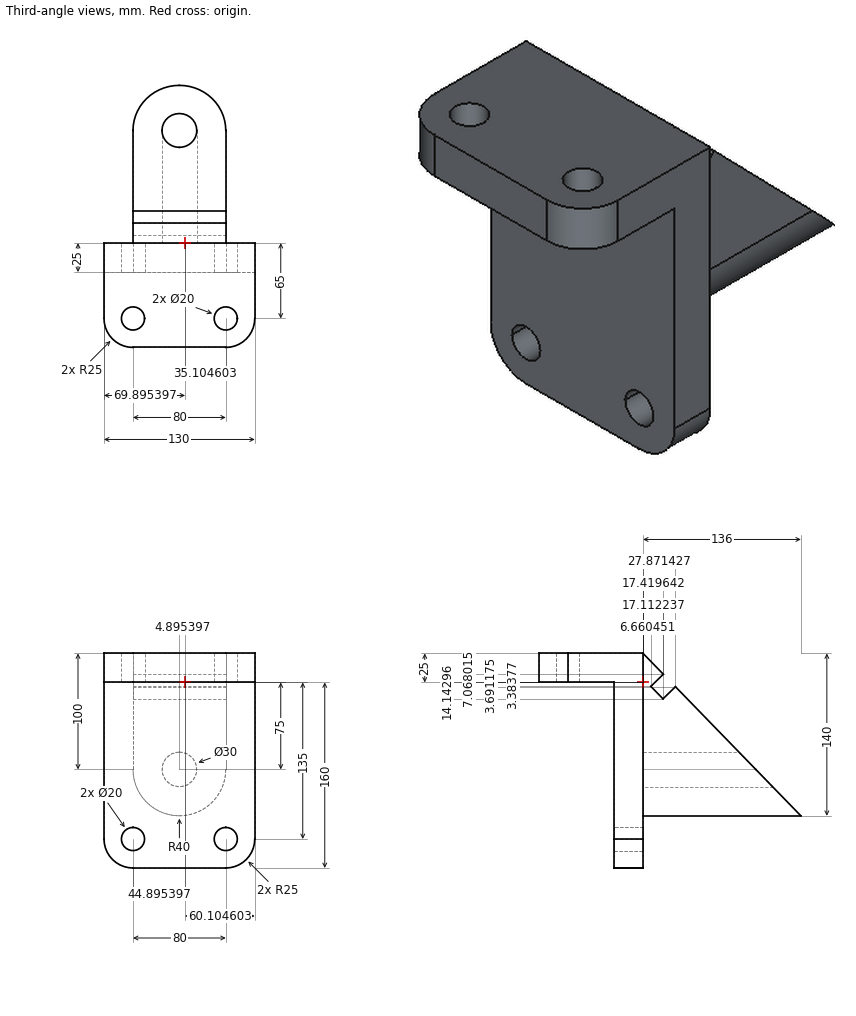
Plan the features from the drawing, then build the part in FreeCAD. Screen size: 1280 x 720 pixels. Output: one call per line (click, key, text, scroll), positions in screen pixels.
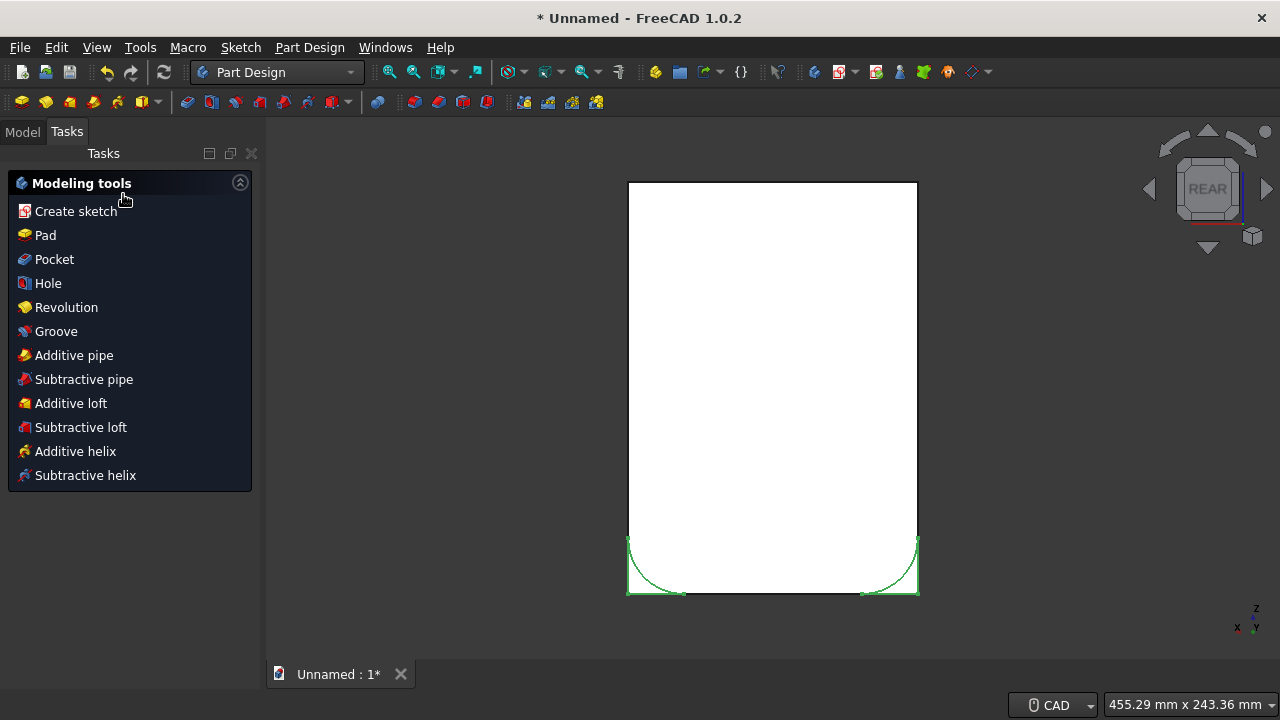
click(188, 102)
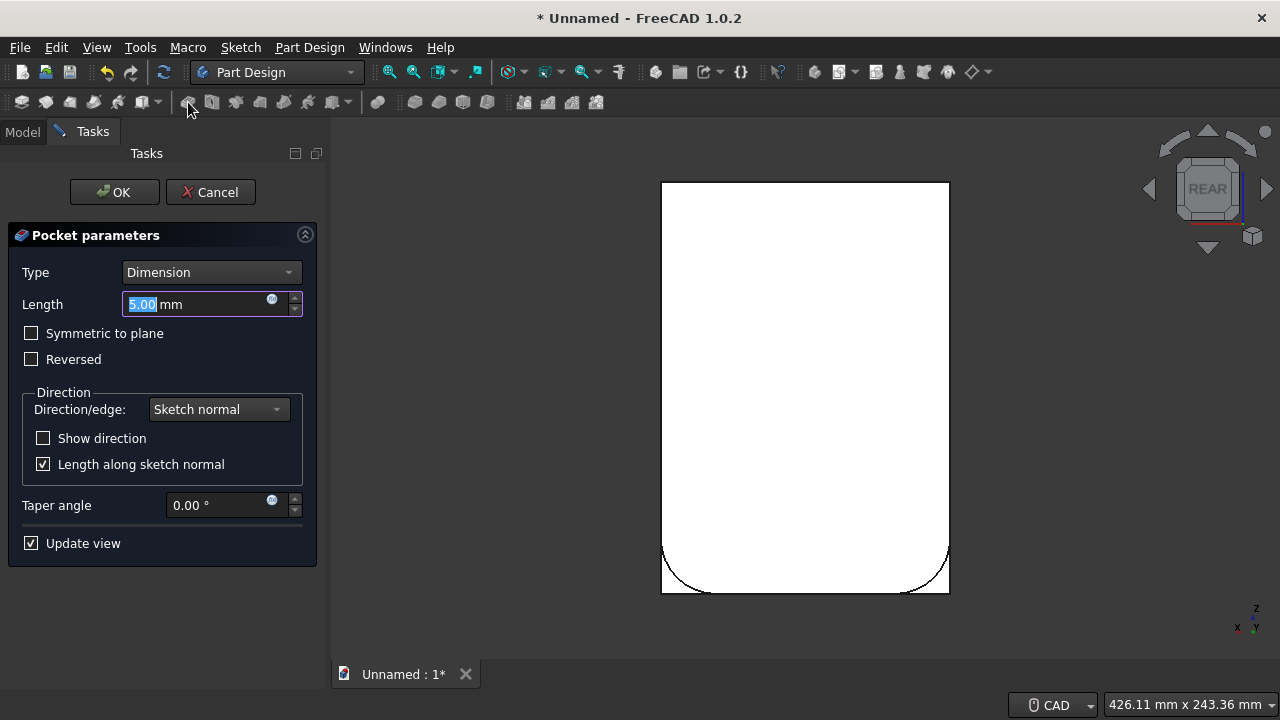
text(160)
key(Tab)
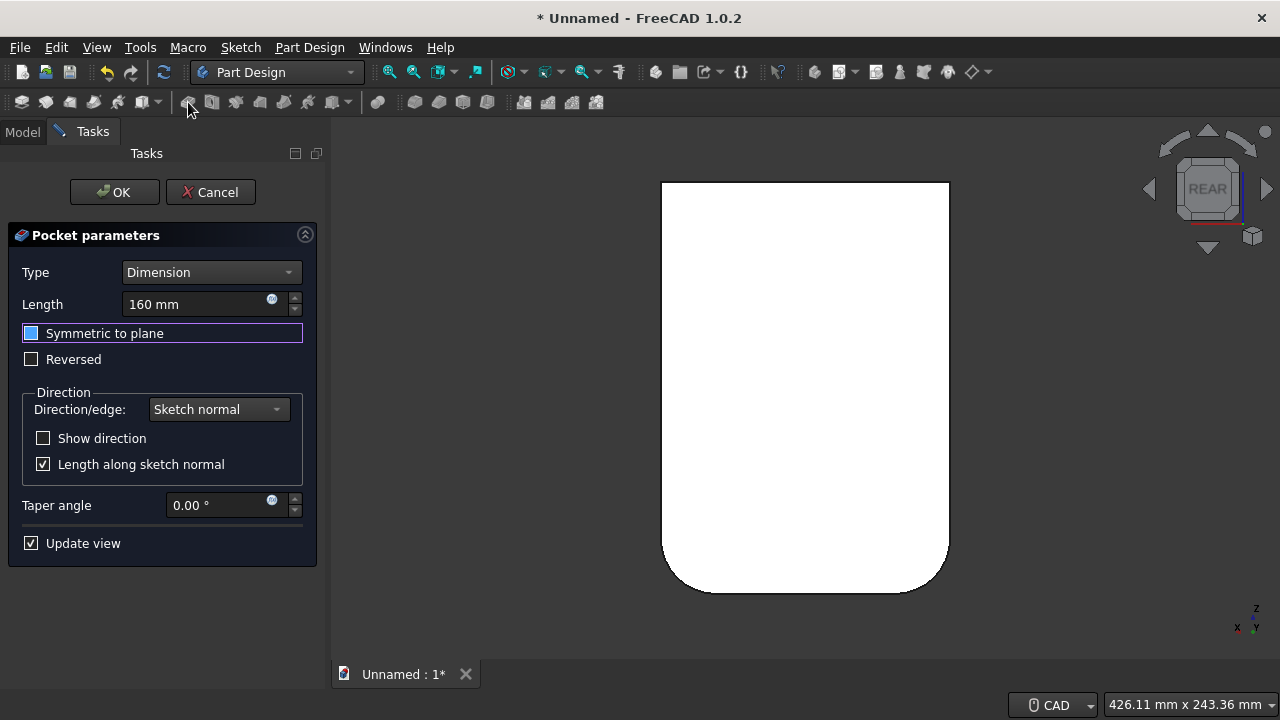
click(115, 192)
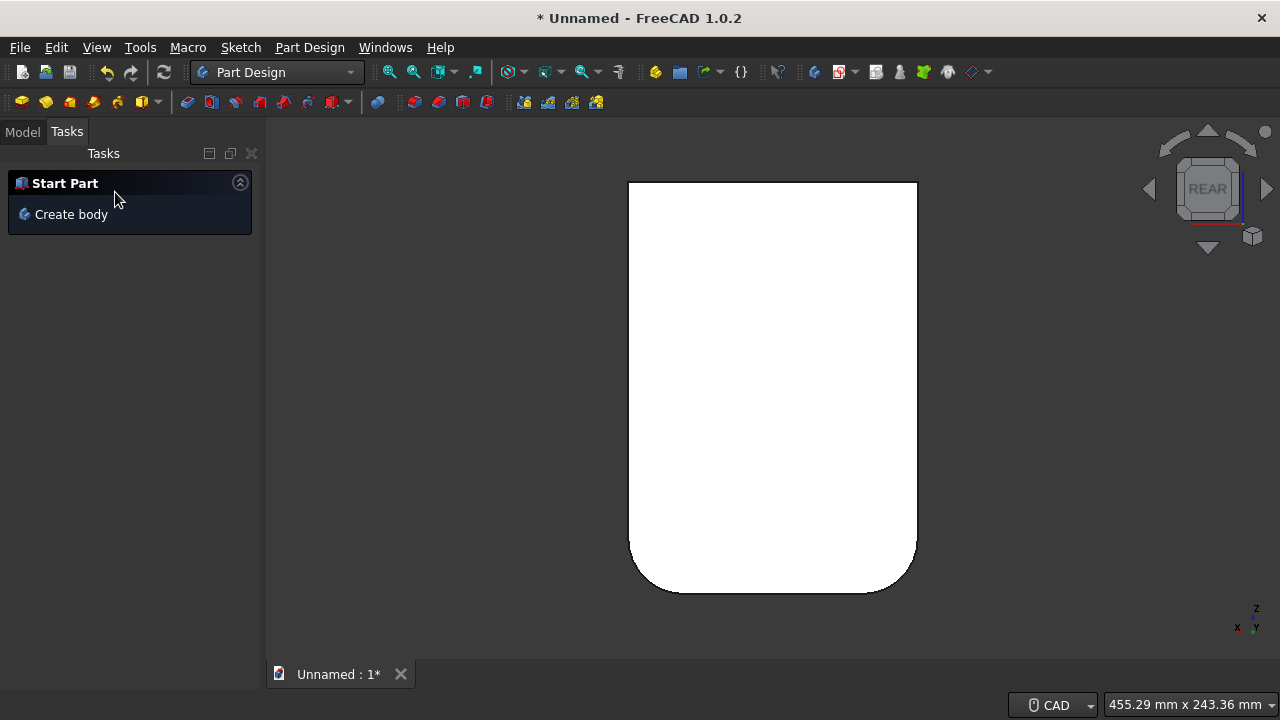
click(773, 328)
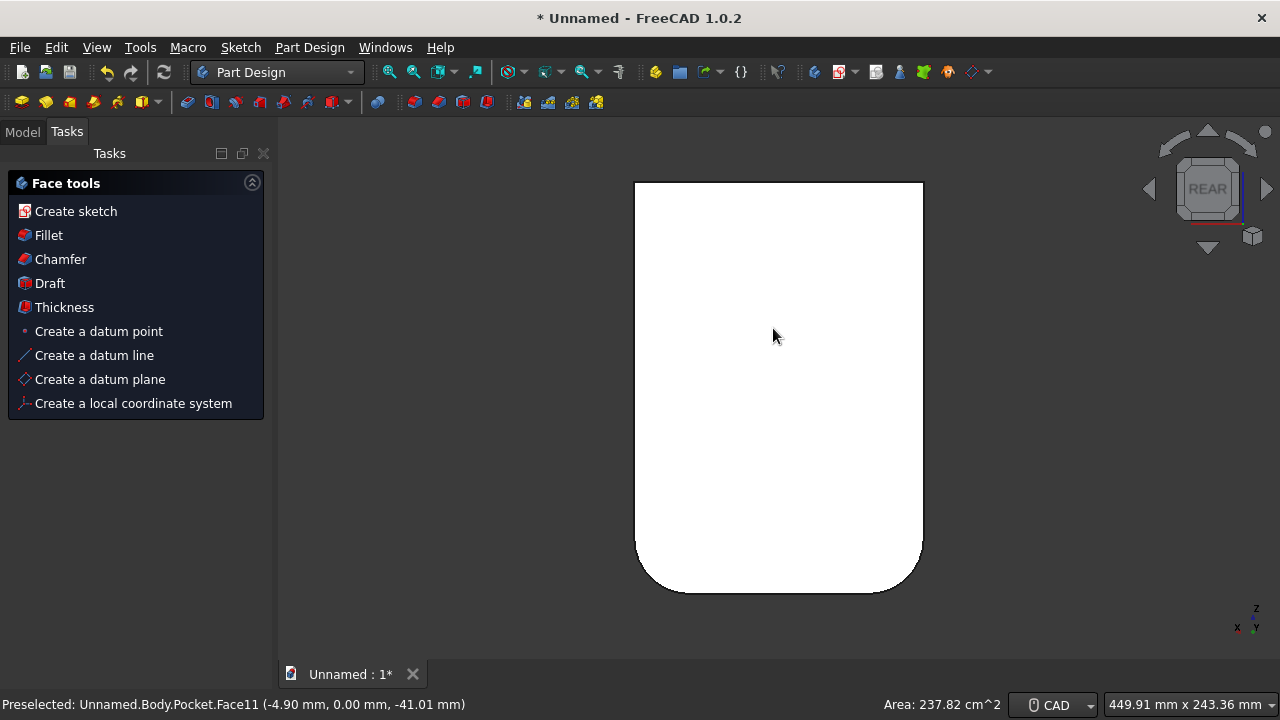
click(840, 72)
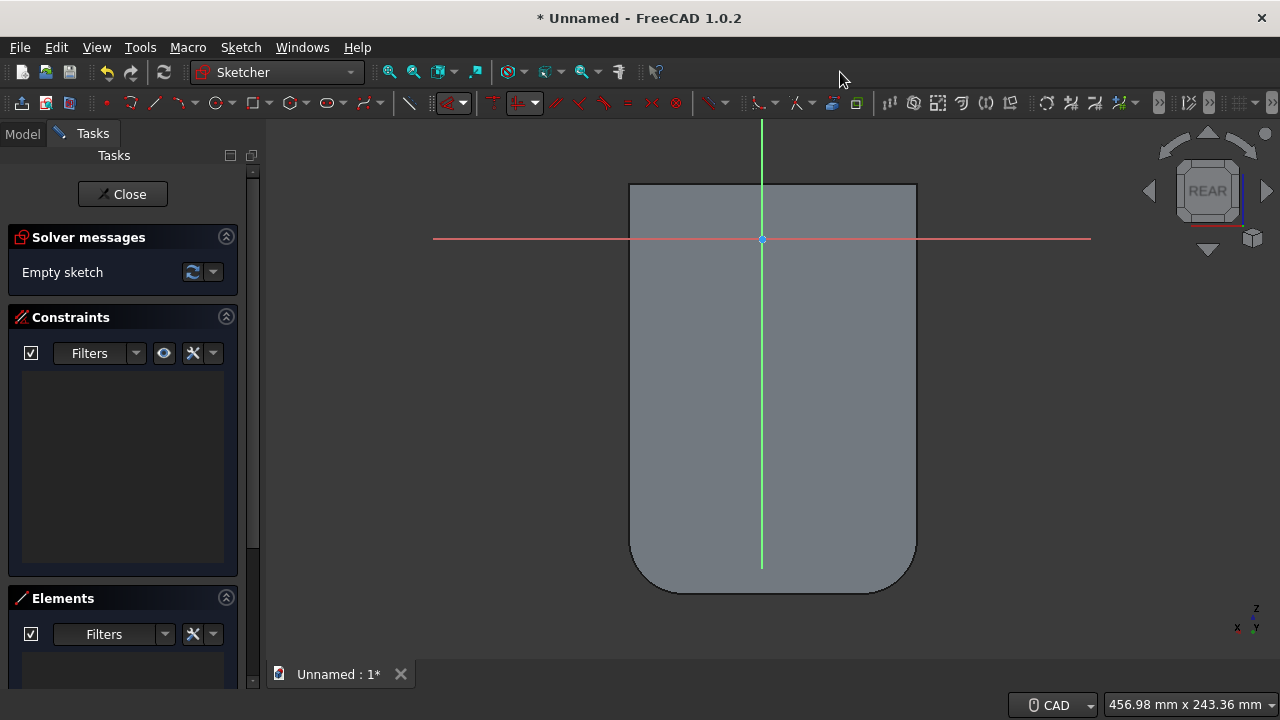
click(216, 104)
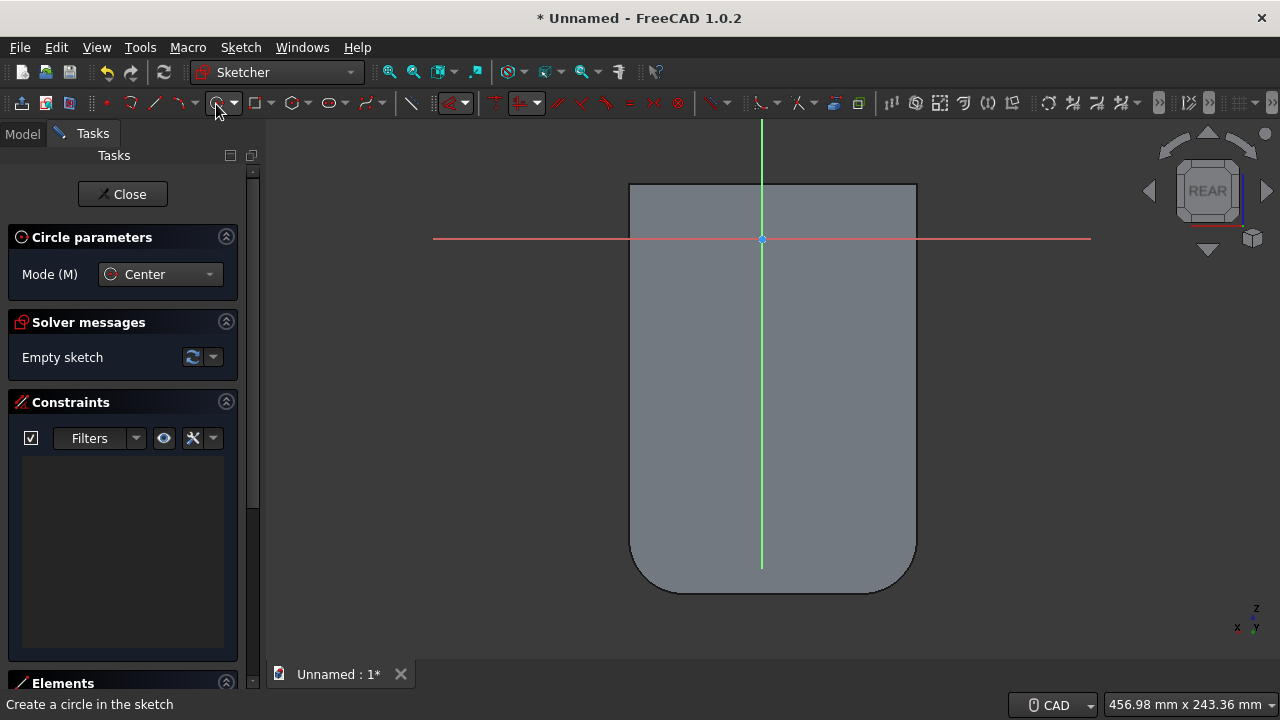
click(862, 539)
click(877, 523)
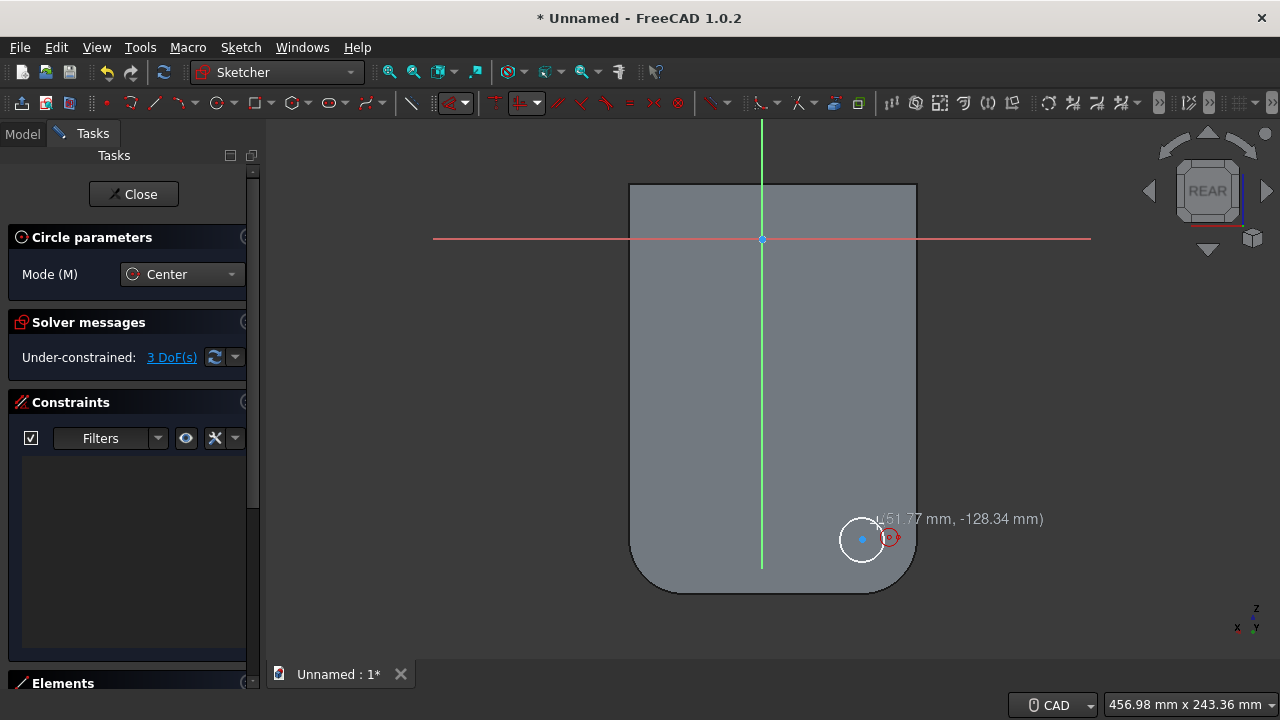
click(684, 539)
click(700, 523)
key(Escape)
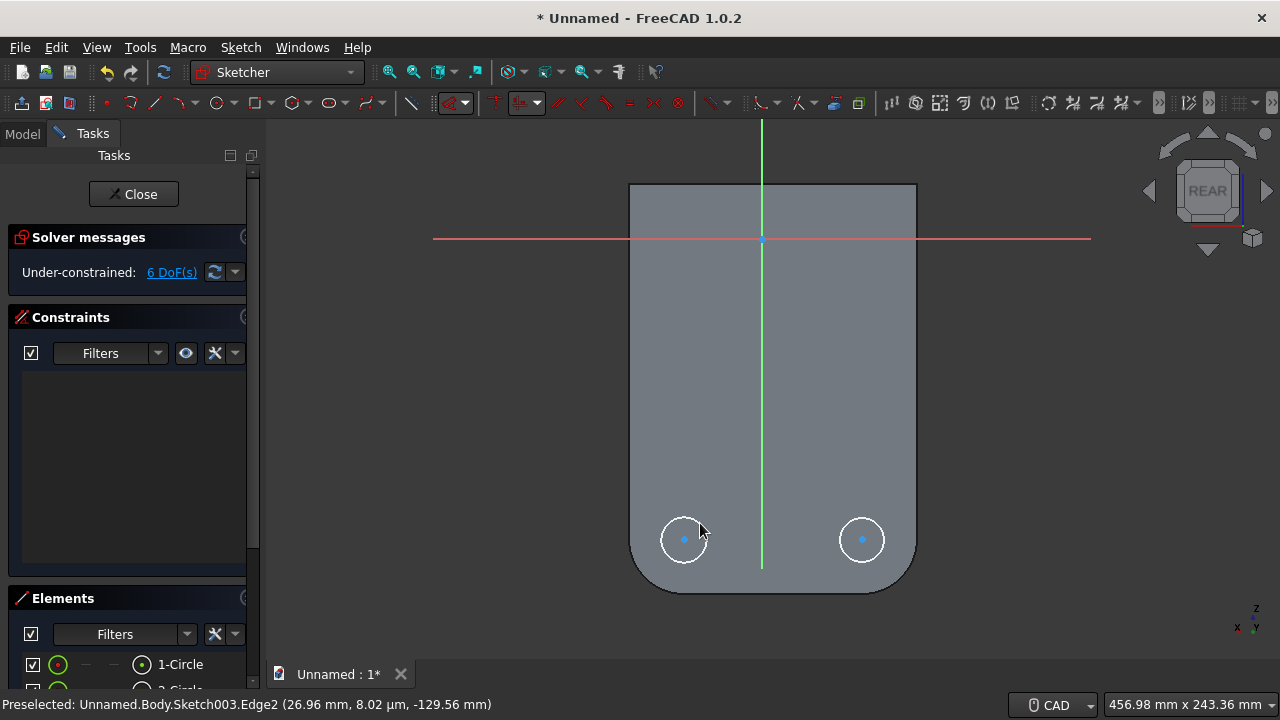
click(877, 524)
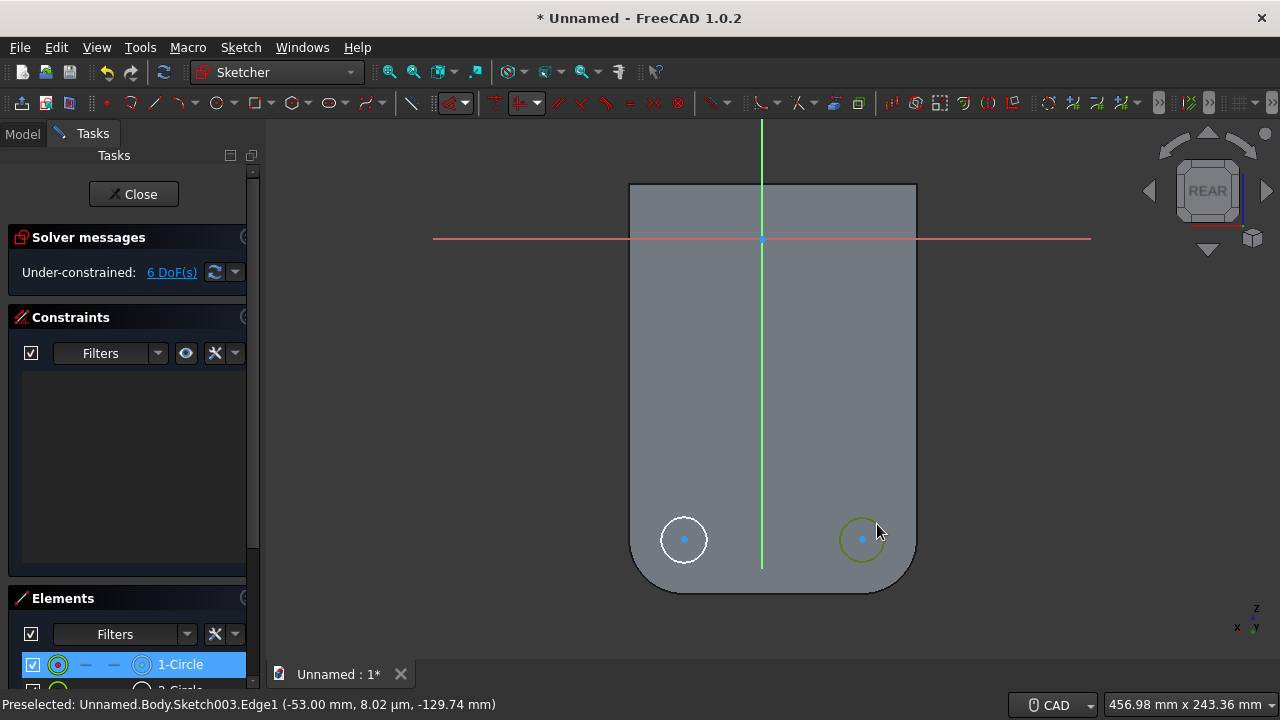
click(700, 524)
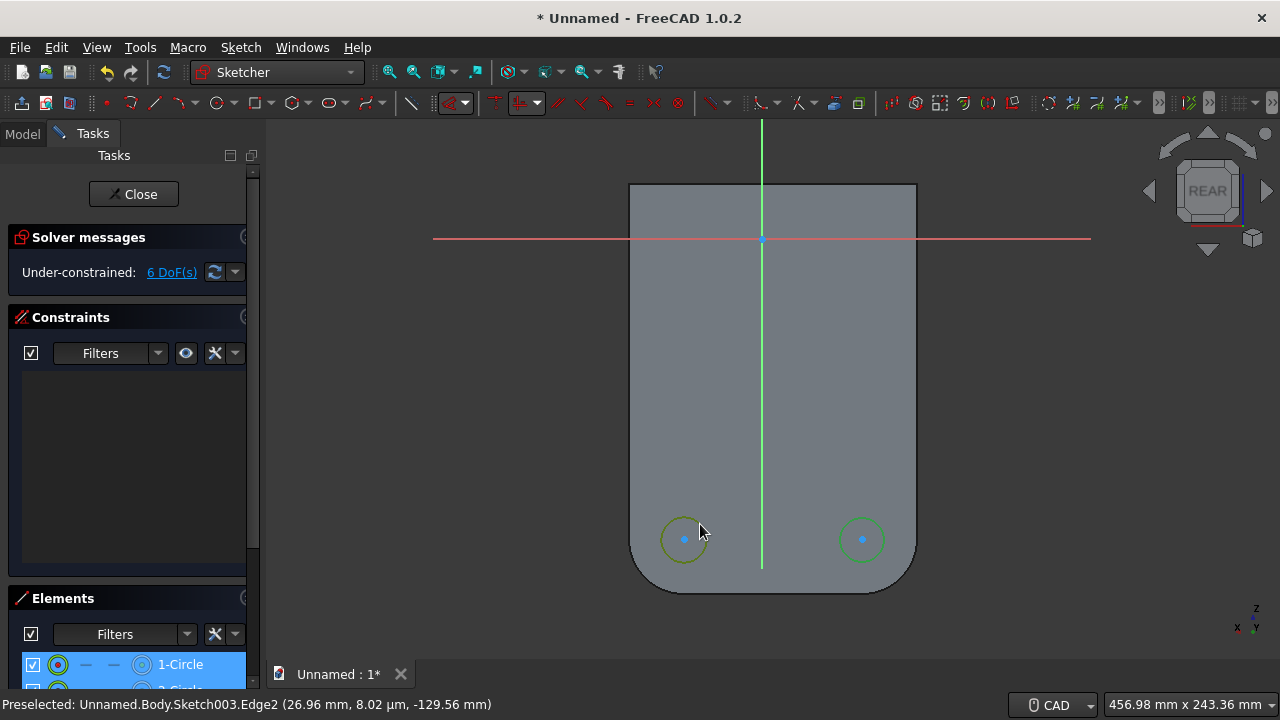
key(e)